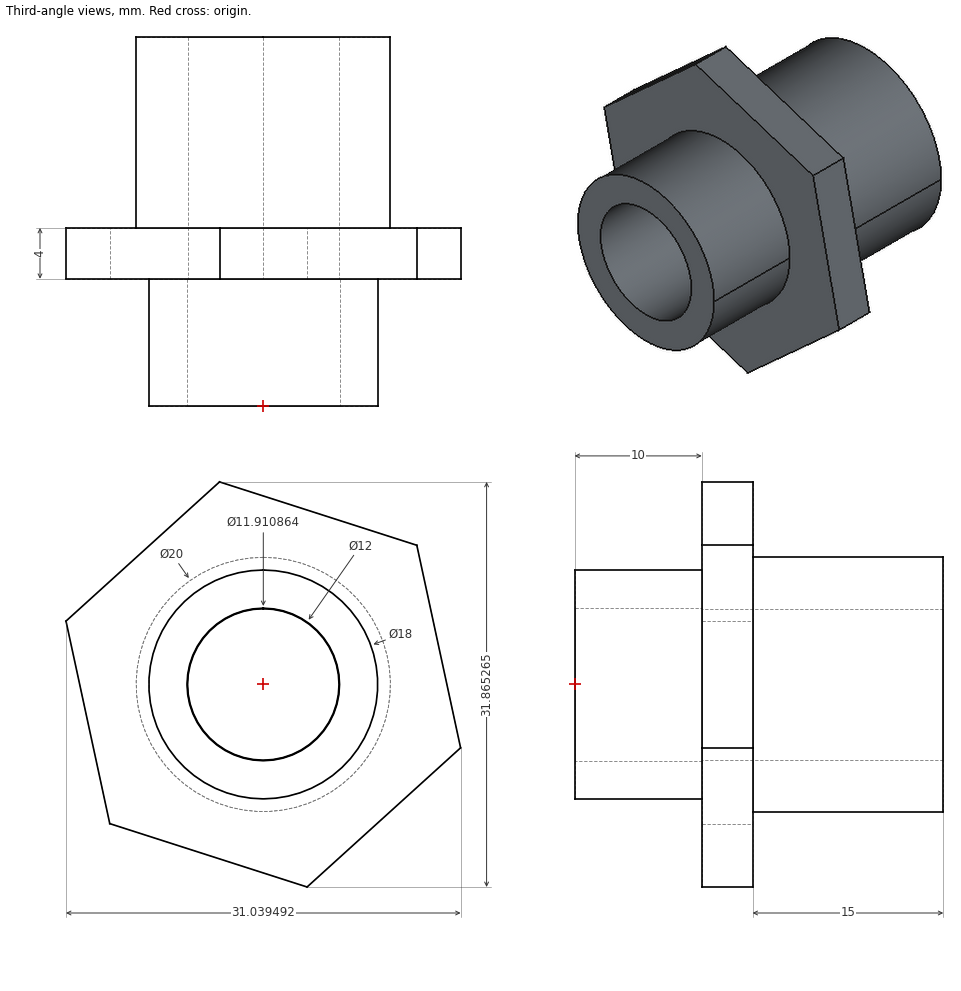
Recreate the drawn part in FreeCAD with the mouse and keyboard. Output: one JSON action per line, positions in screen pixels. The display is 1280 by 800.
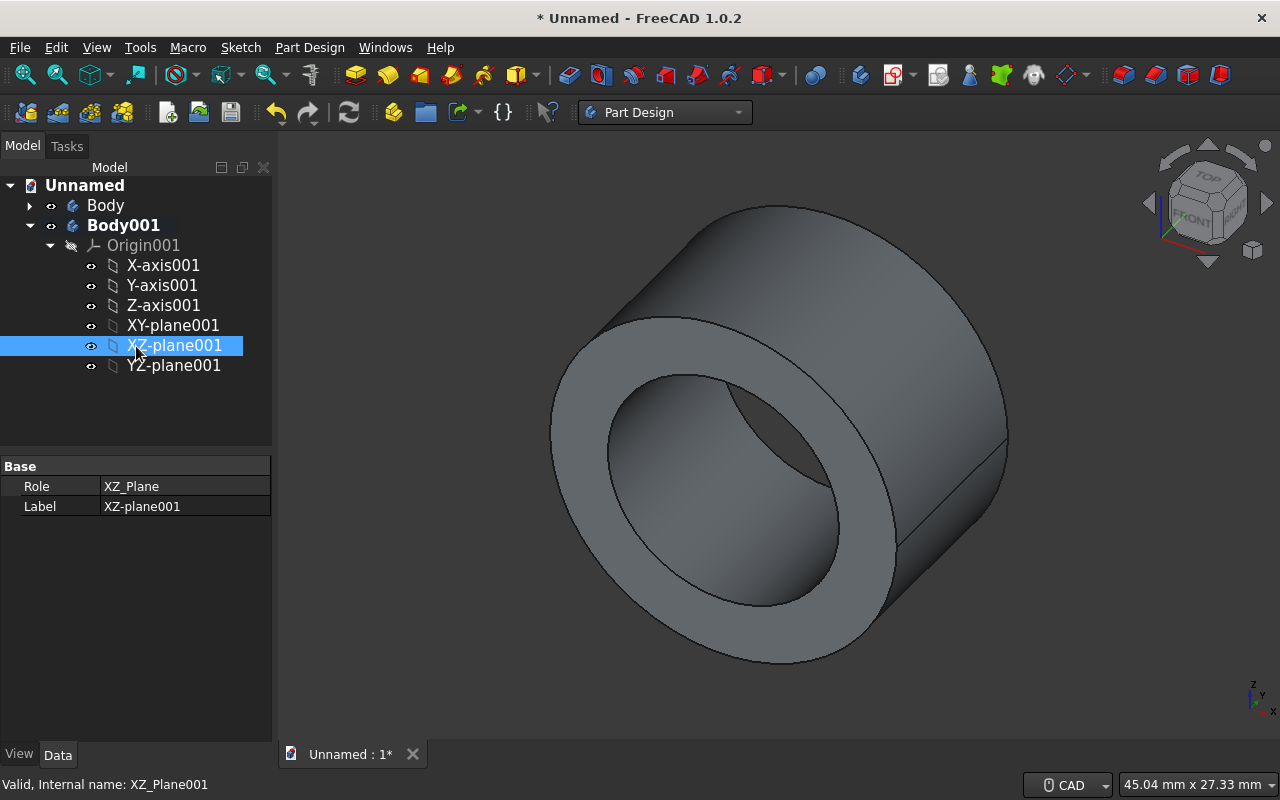
{"action": "left_click", "coordinate": [1066, 76]}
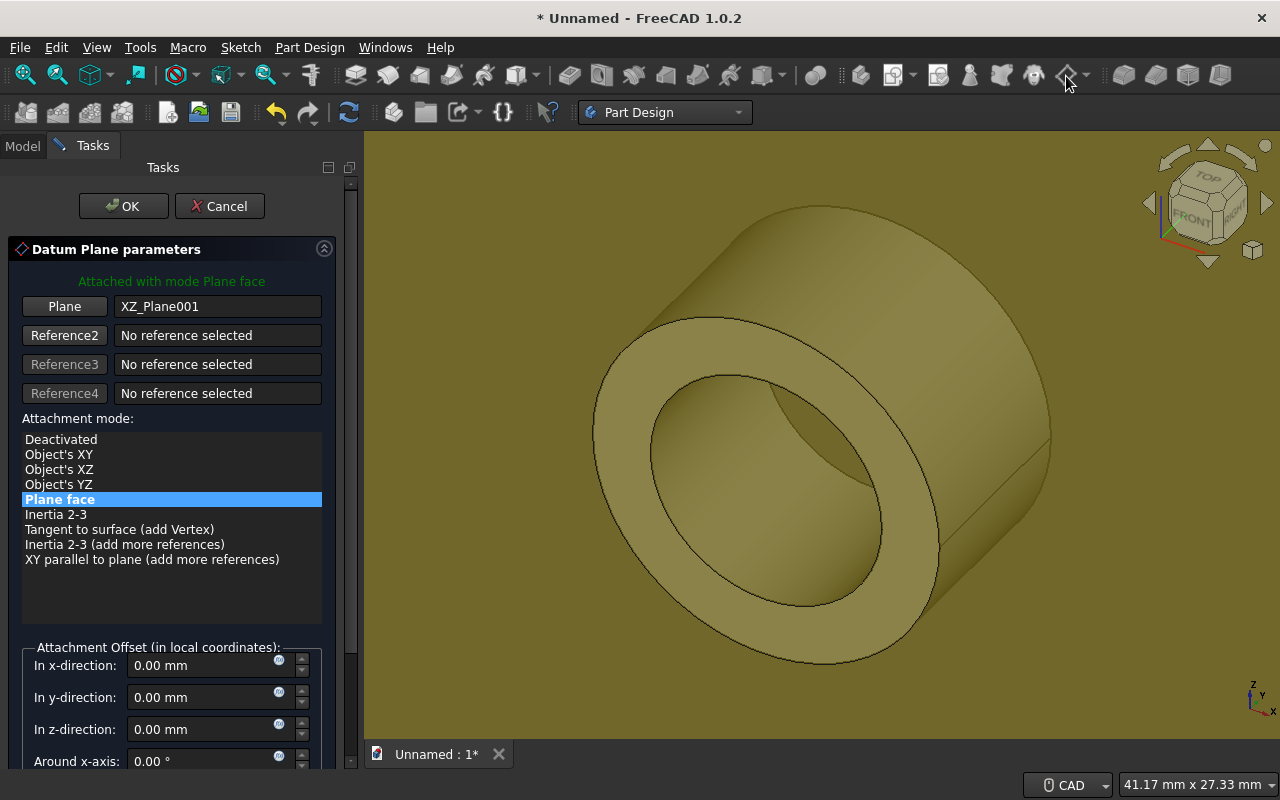
{"action": "triple_click", "coordinate": [210, 729]}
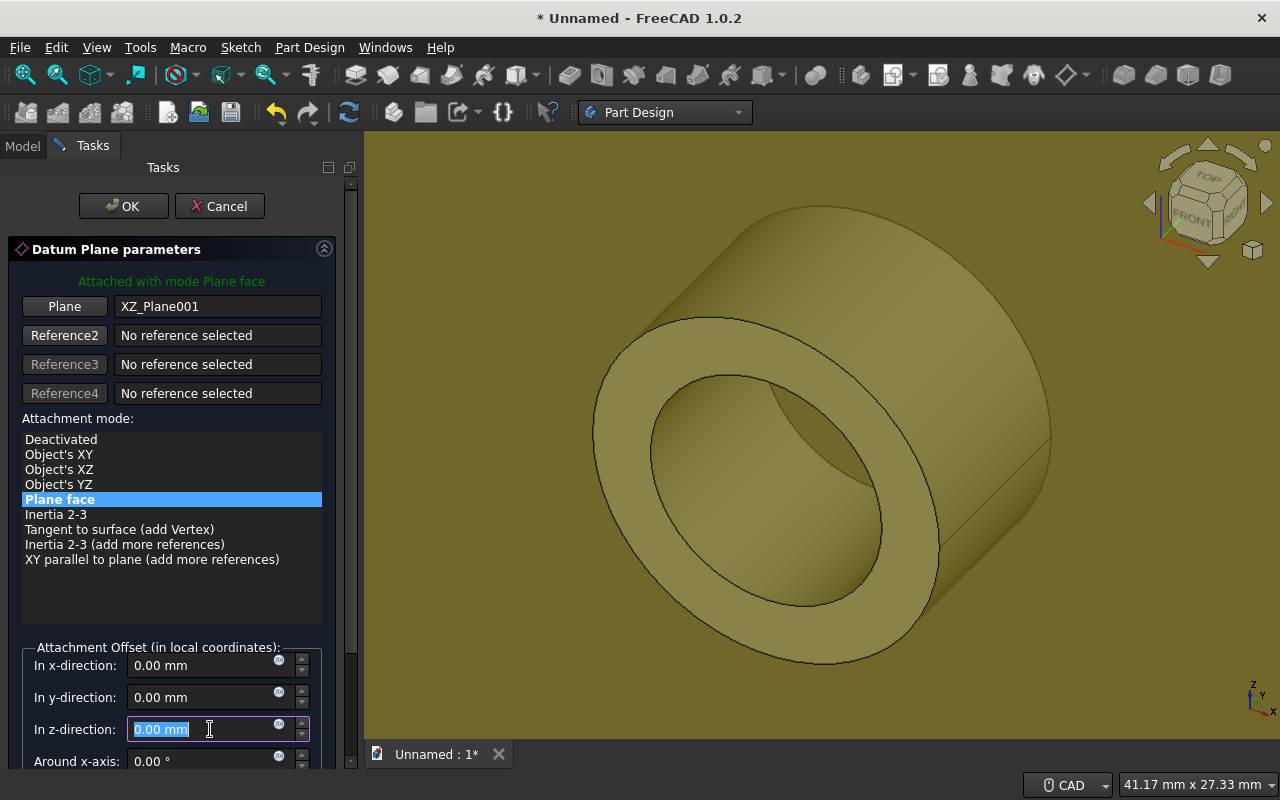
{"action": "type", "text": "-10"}
{"action": "key", "text": "Tab"}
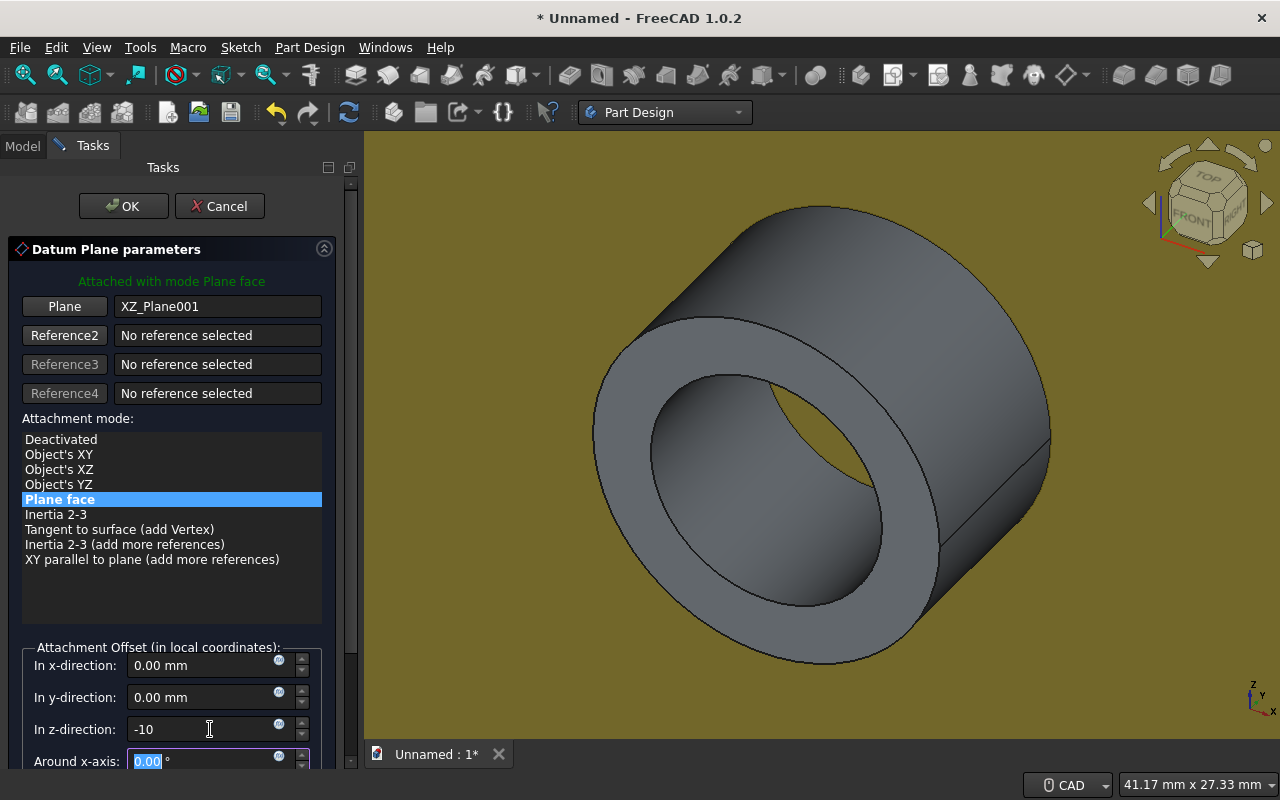
{"action": "left_click", "coordinate": [124, 206]}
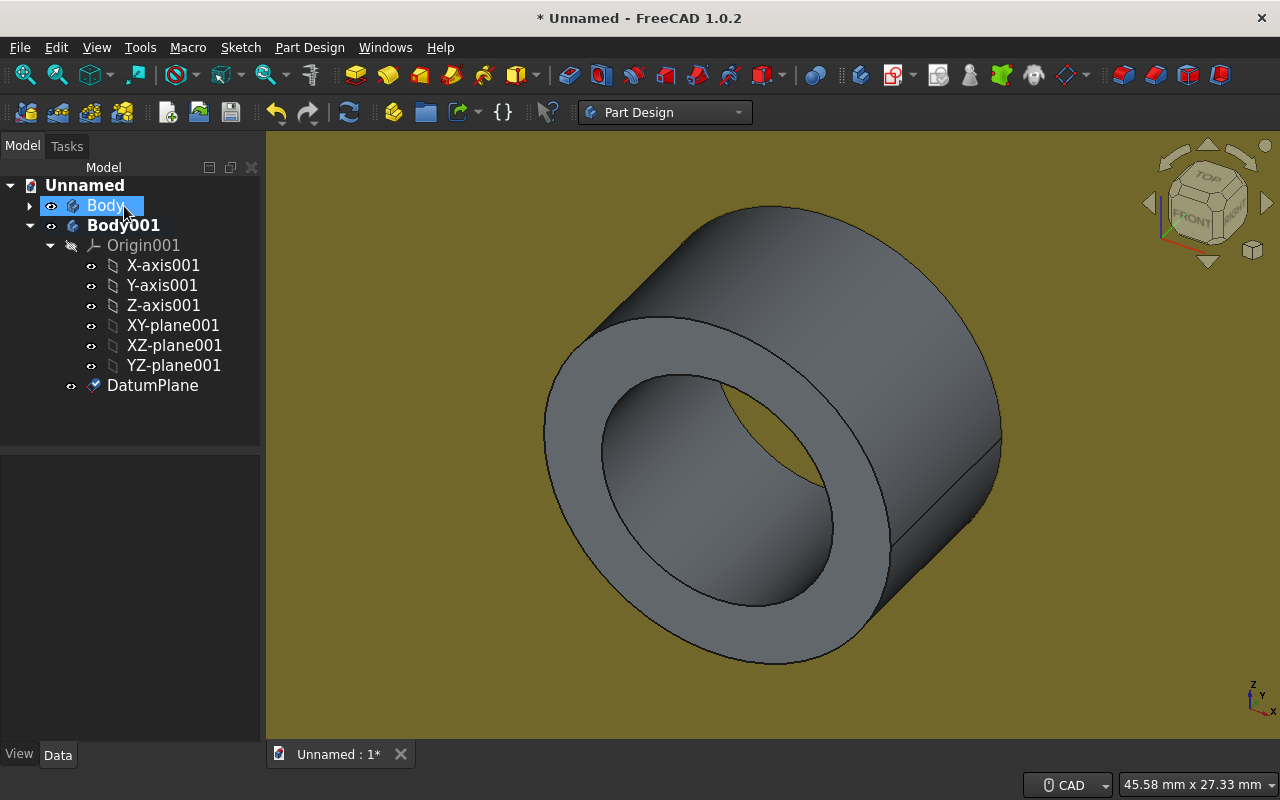
{"action": "left_click", "coordinate": [116, 386]}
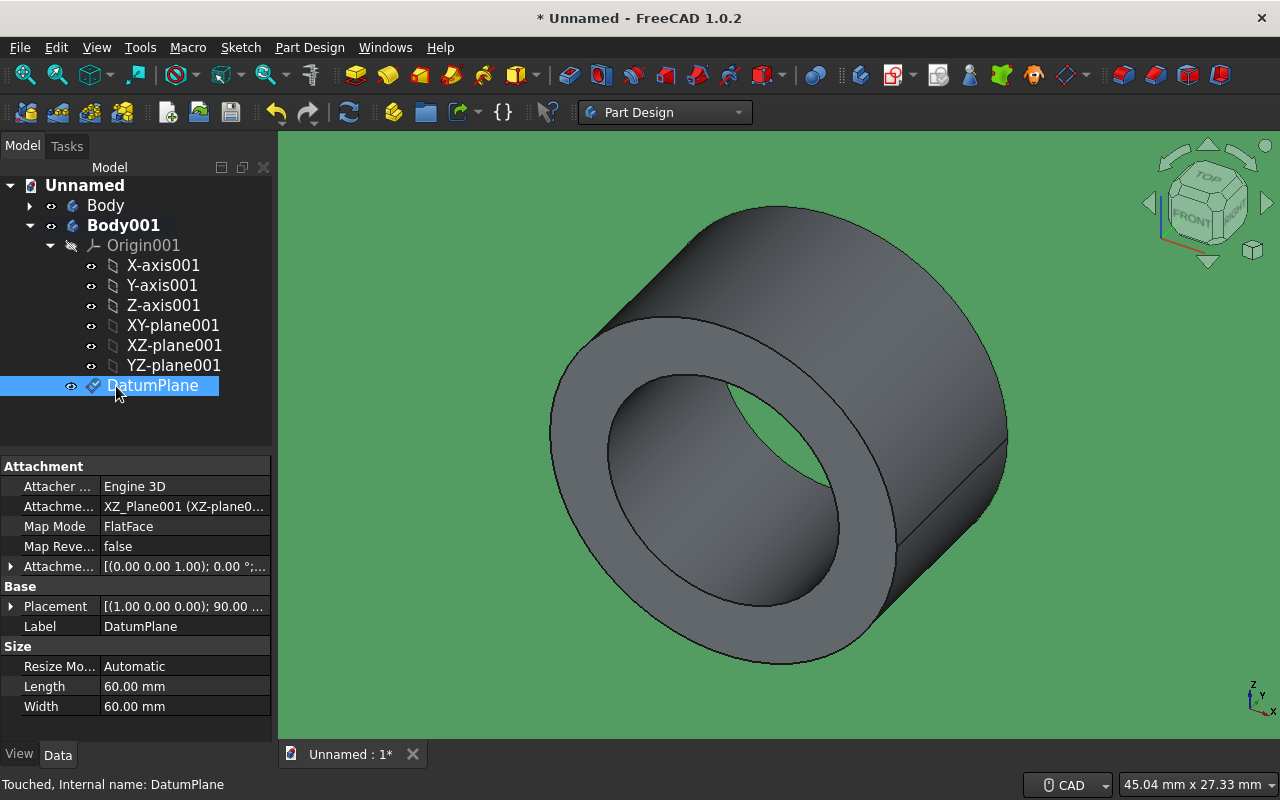
{"action": "left_click", "coordinate": [894, 76]}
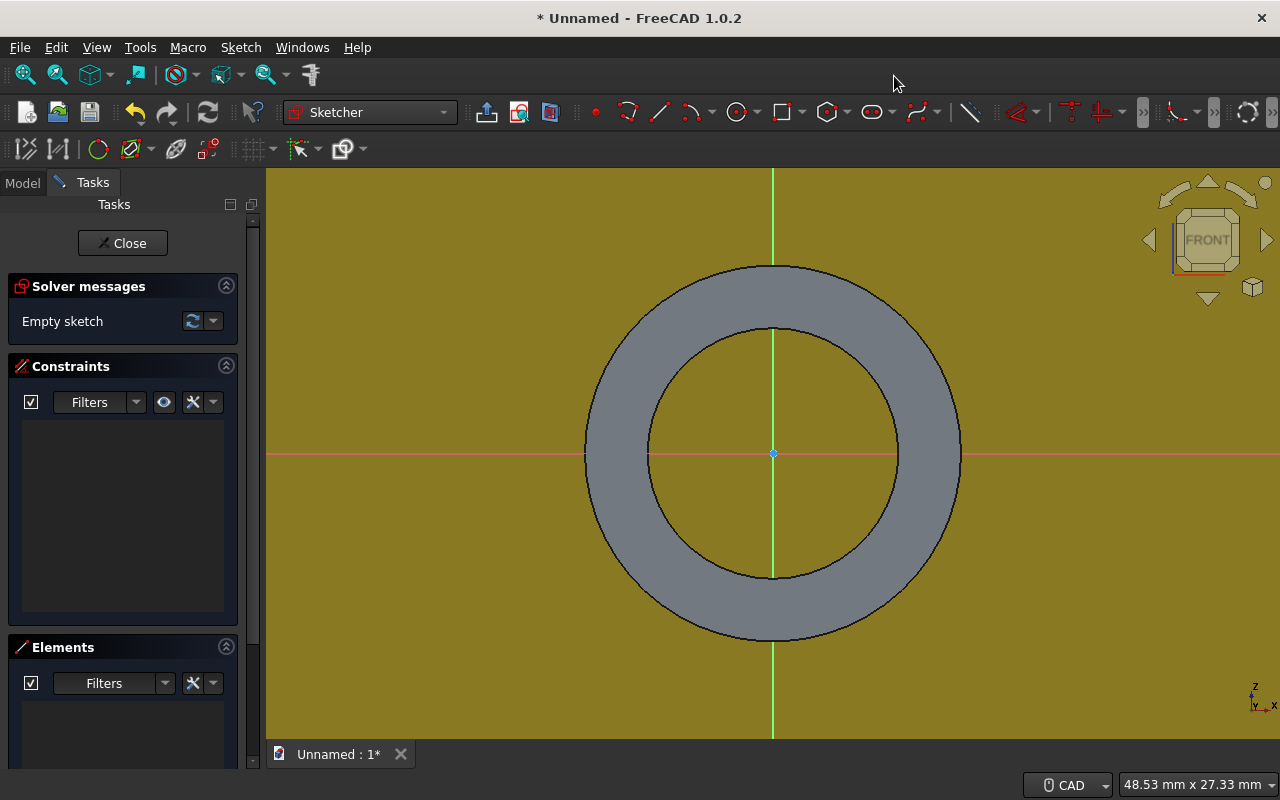
{"action": "scroll", "coordinate": [621, 453], "scroll_direction": "down", "scroll_amount": 3}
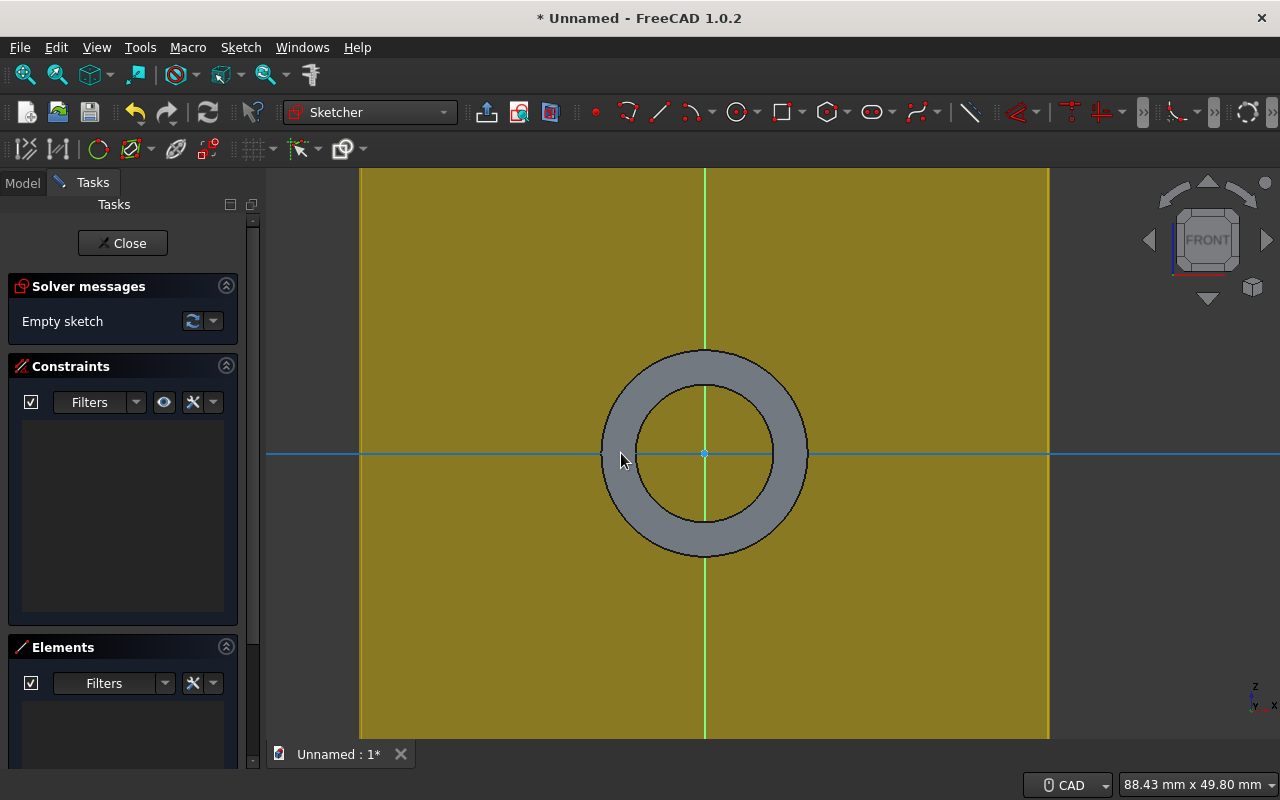
{"action": "left_click", "coordinate": [828, 112]}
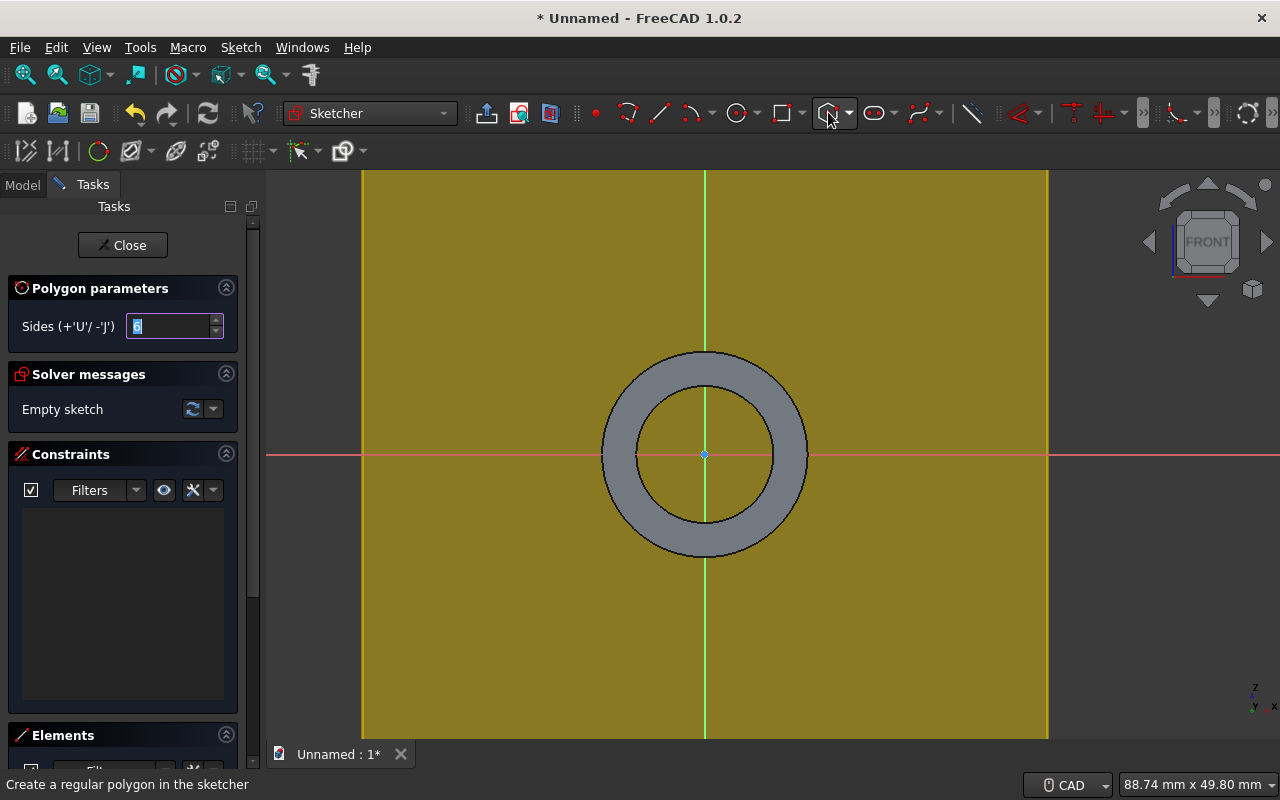
{"action": "left_click", "coordinate": [705, 455]}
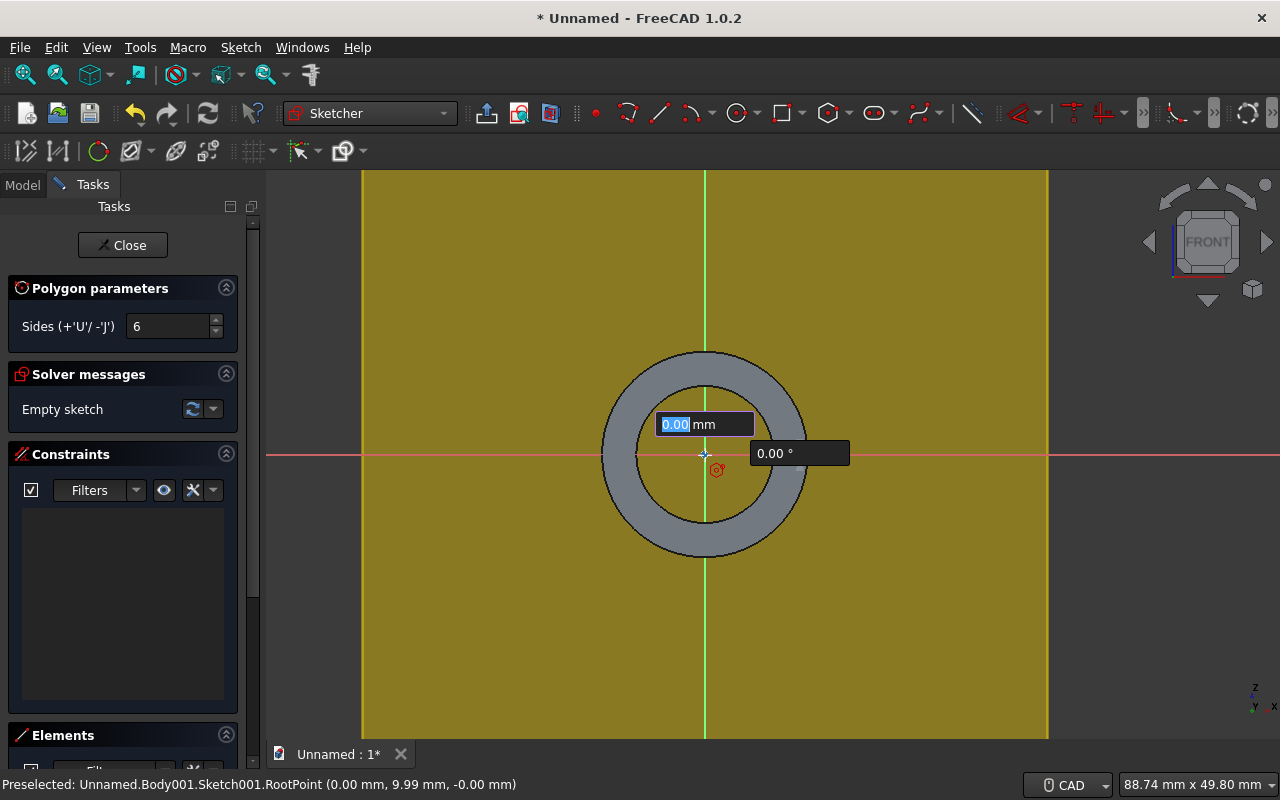
{"action": "left_click", "coordinate": [567, 580]}
{"action": "right_click", "coordinate": [567, 580]}